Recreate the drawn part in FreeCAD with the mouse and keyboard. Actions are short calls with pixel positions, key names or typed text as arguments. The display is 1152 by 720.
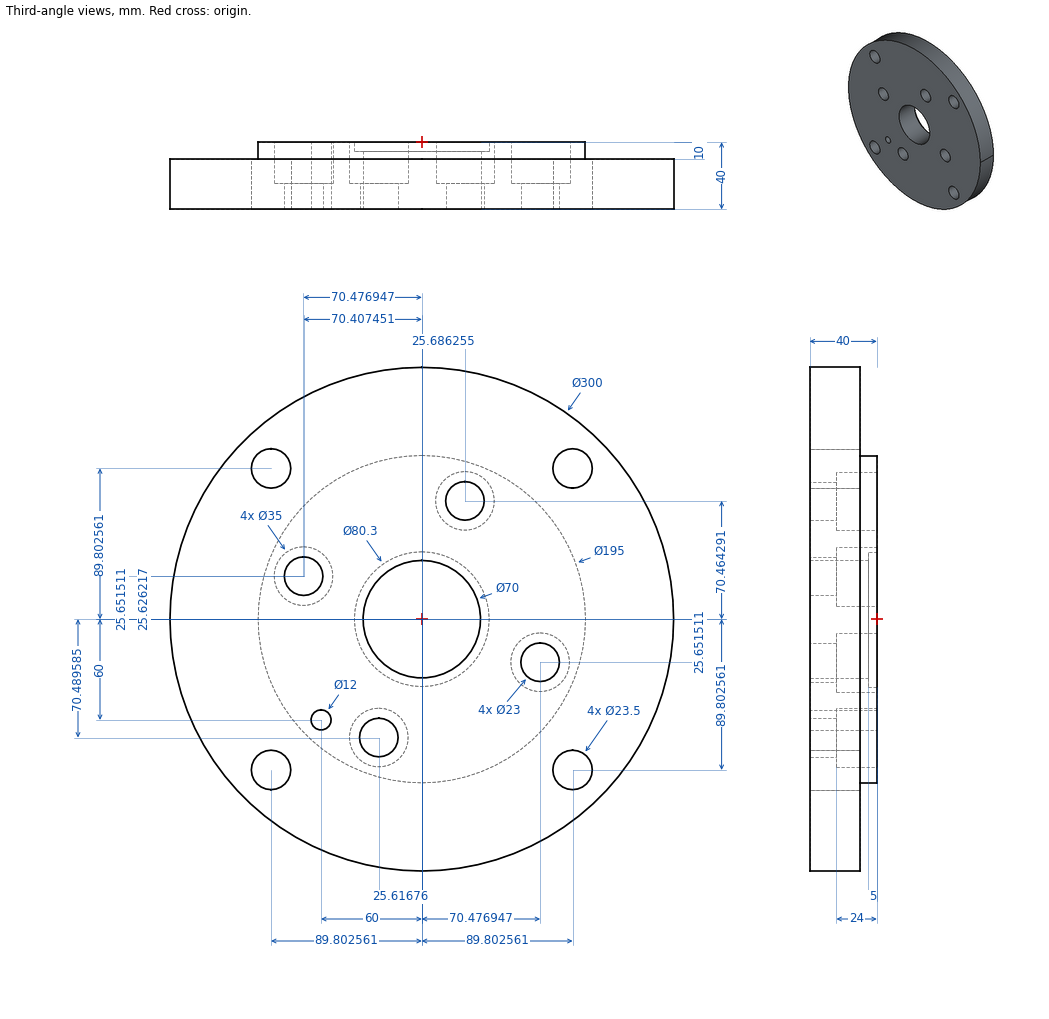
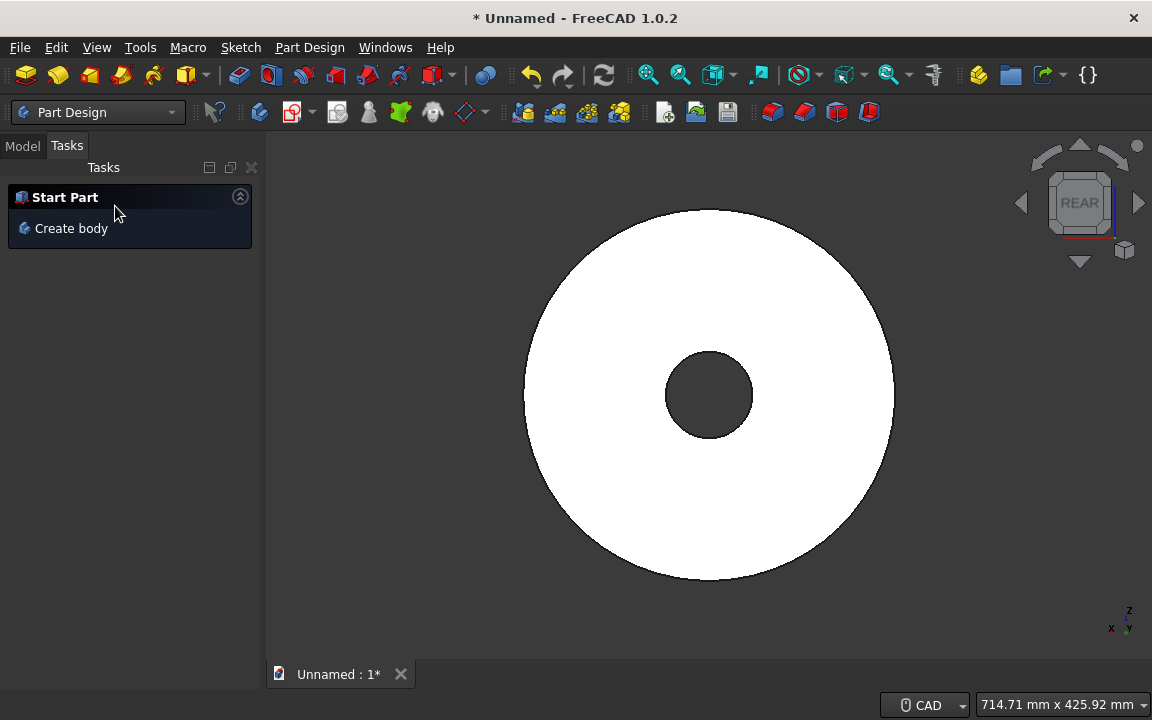
click(656, 500)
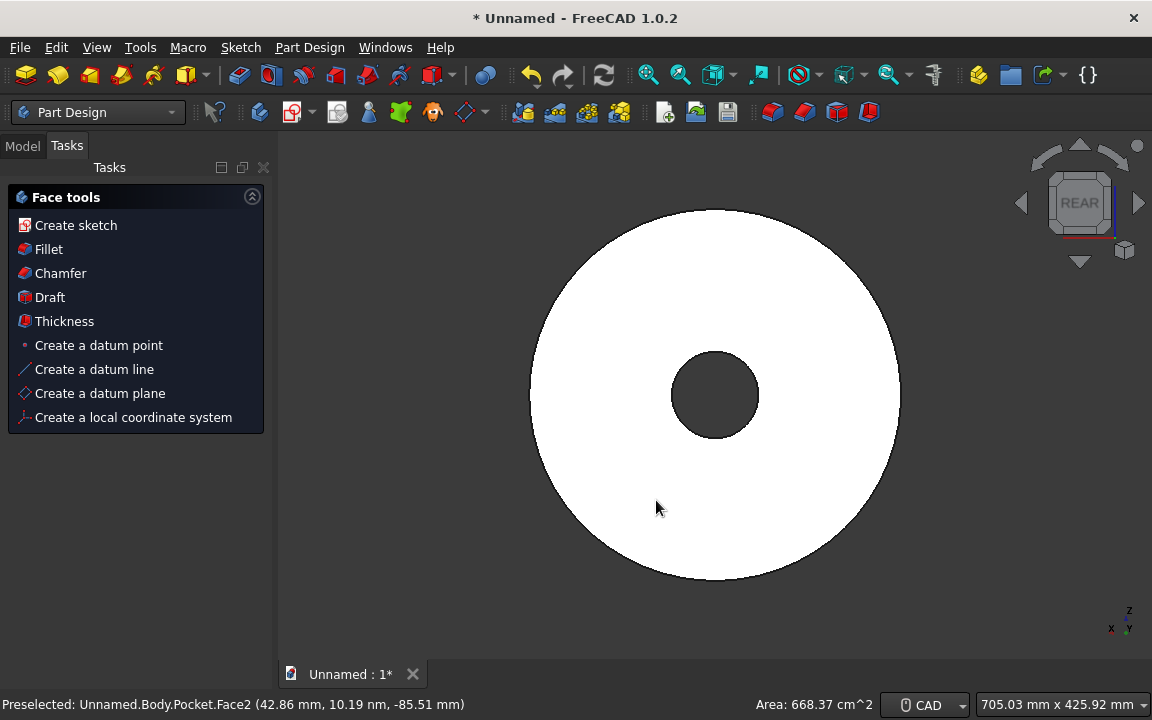
click(292, 112)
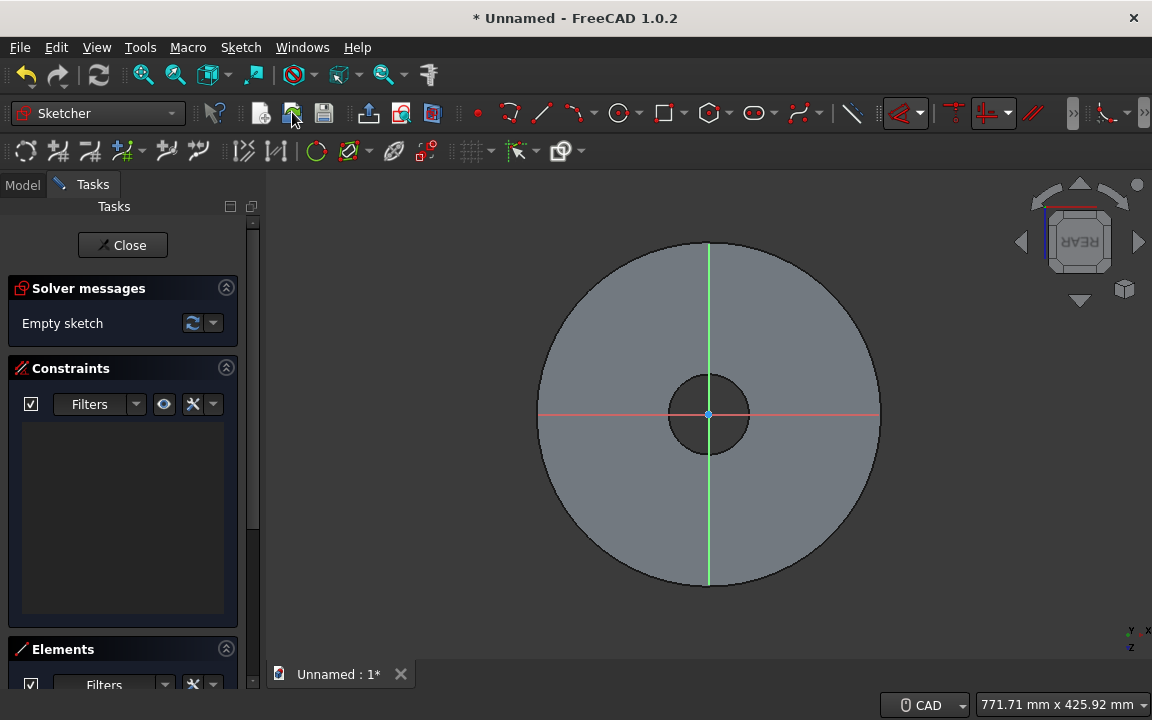
scroll(738, 414, up, 6)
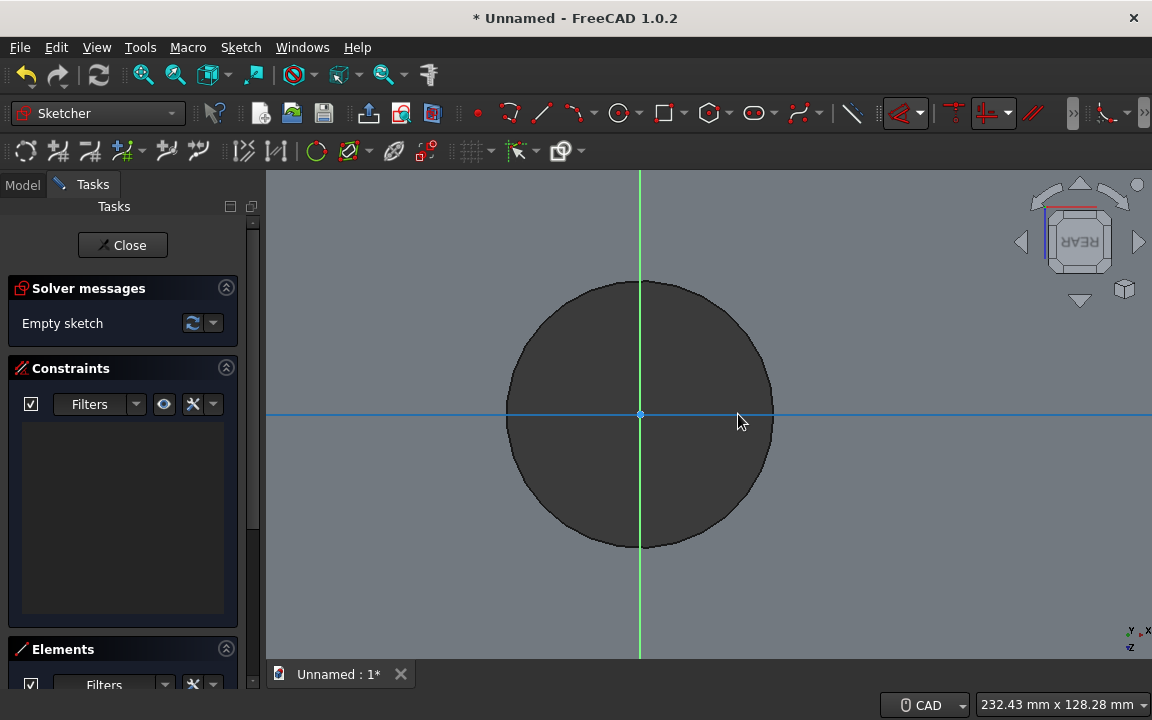
click(620, 114)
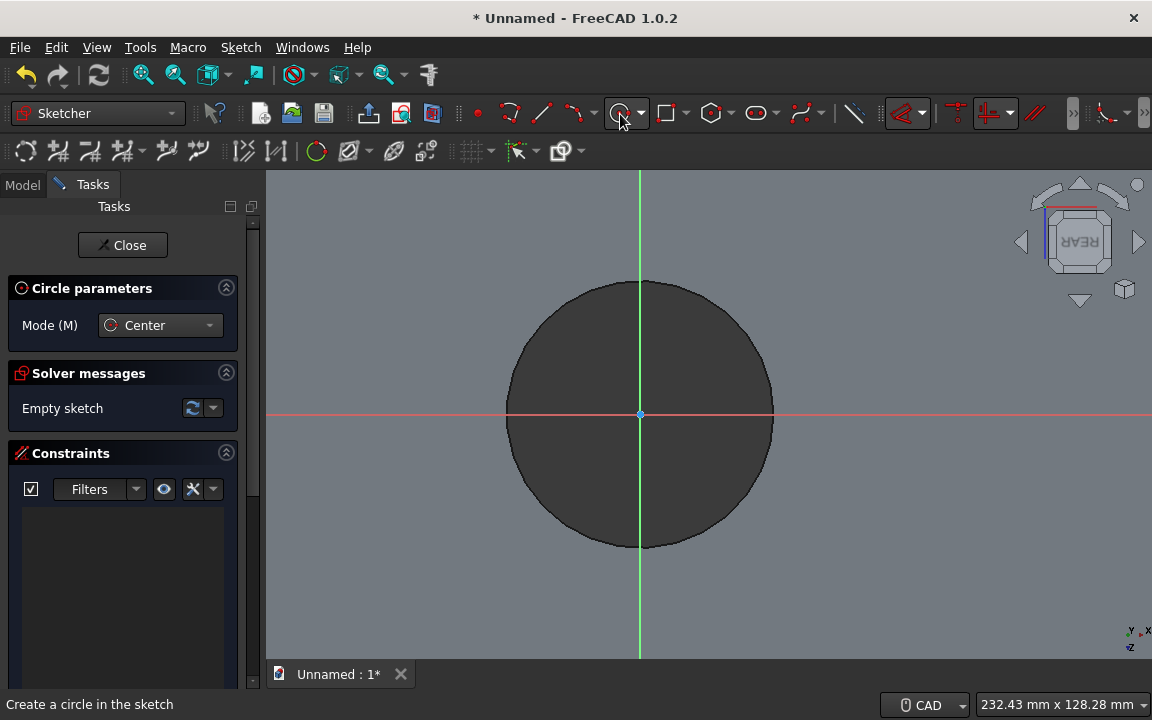
click(640, 414)
move(748, 306)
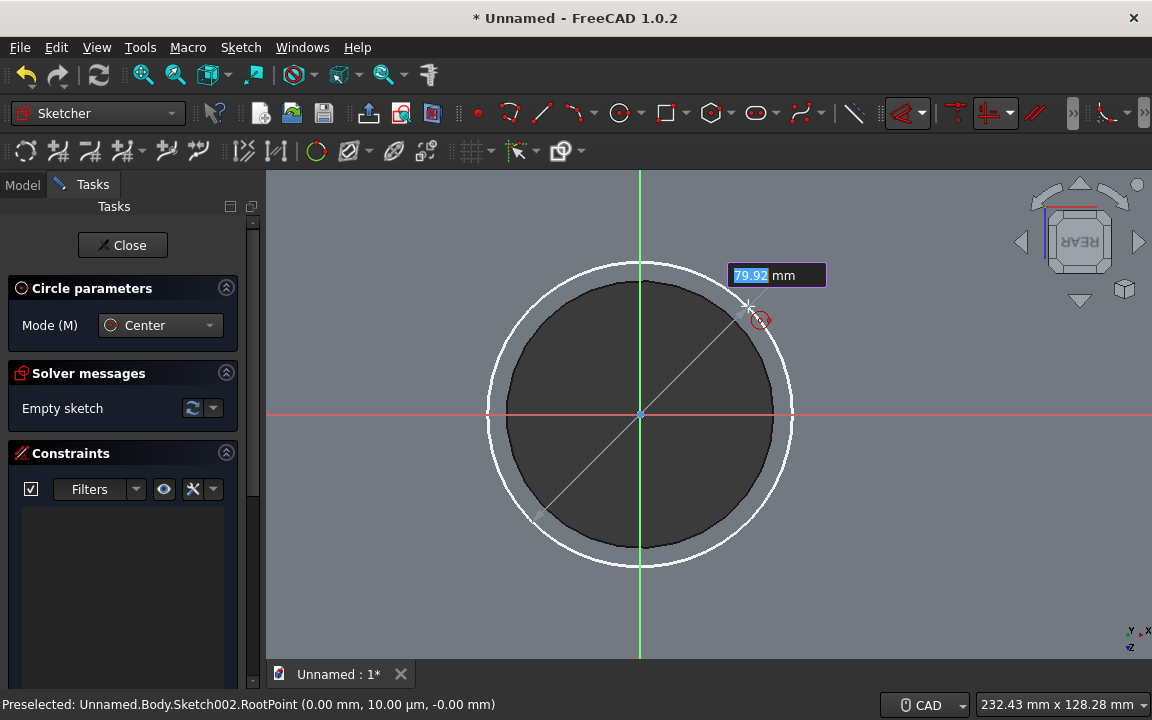
text(80.3)
key(Return)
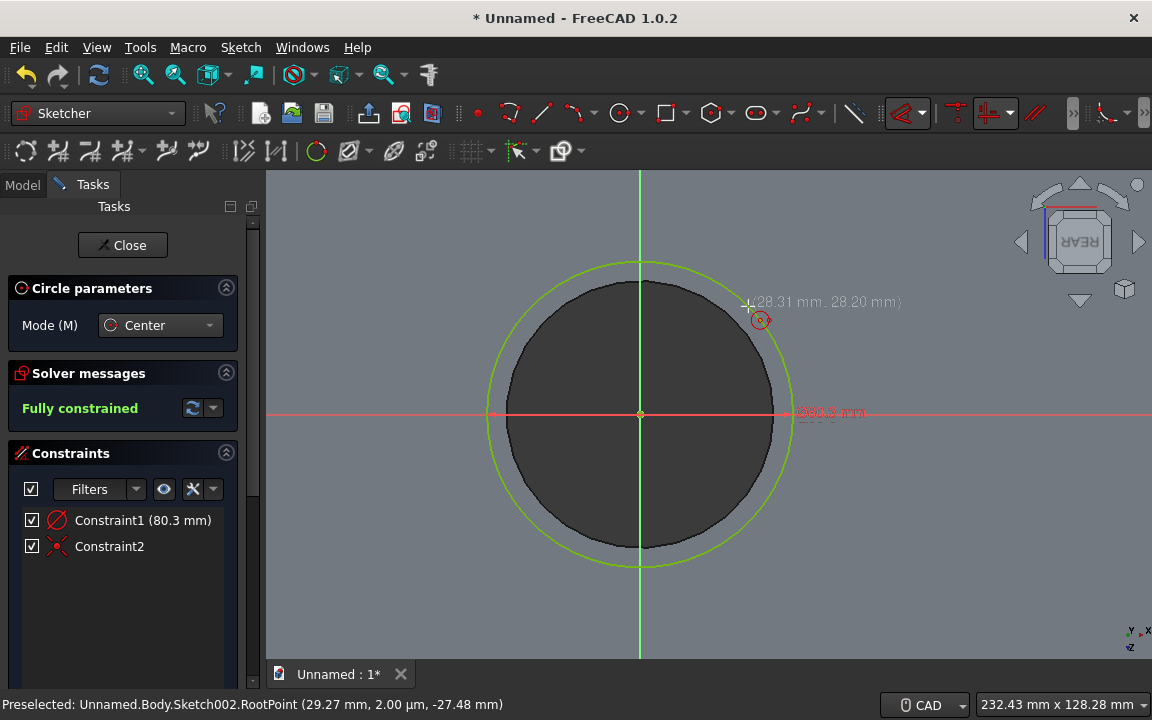
click(640, 414)
move(734, 320)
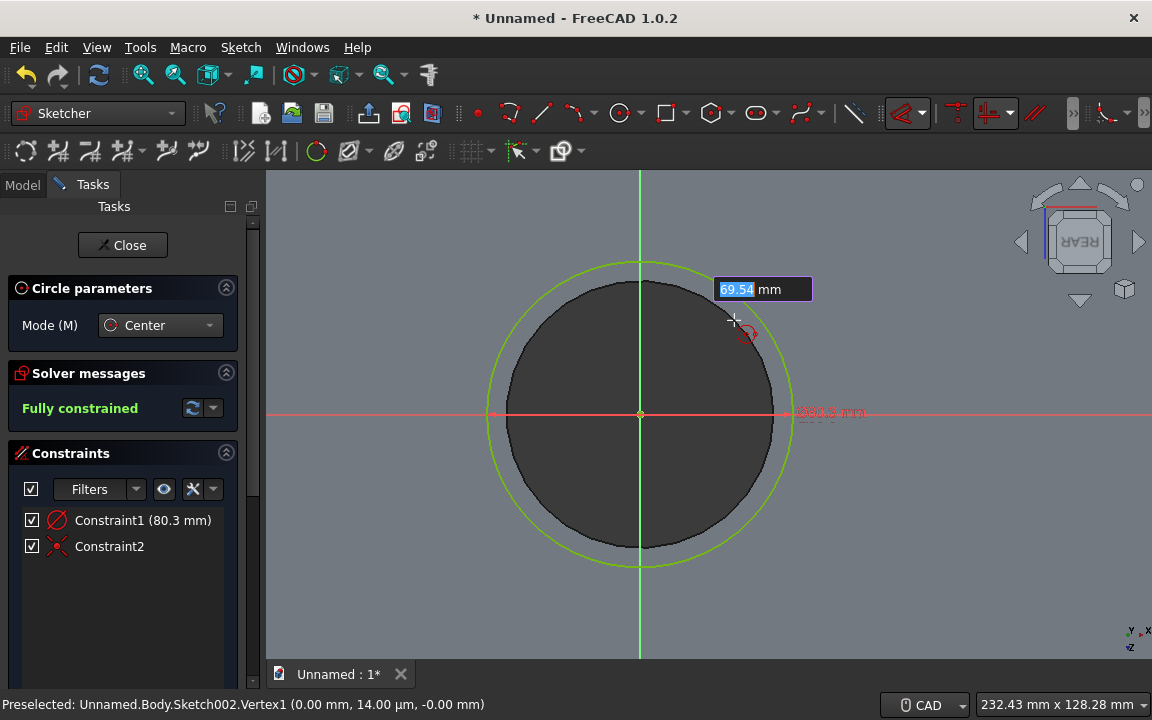
text(70)
key(Return)
key(Escape)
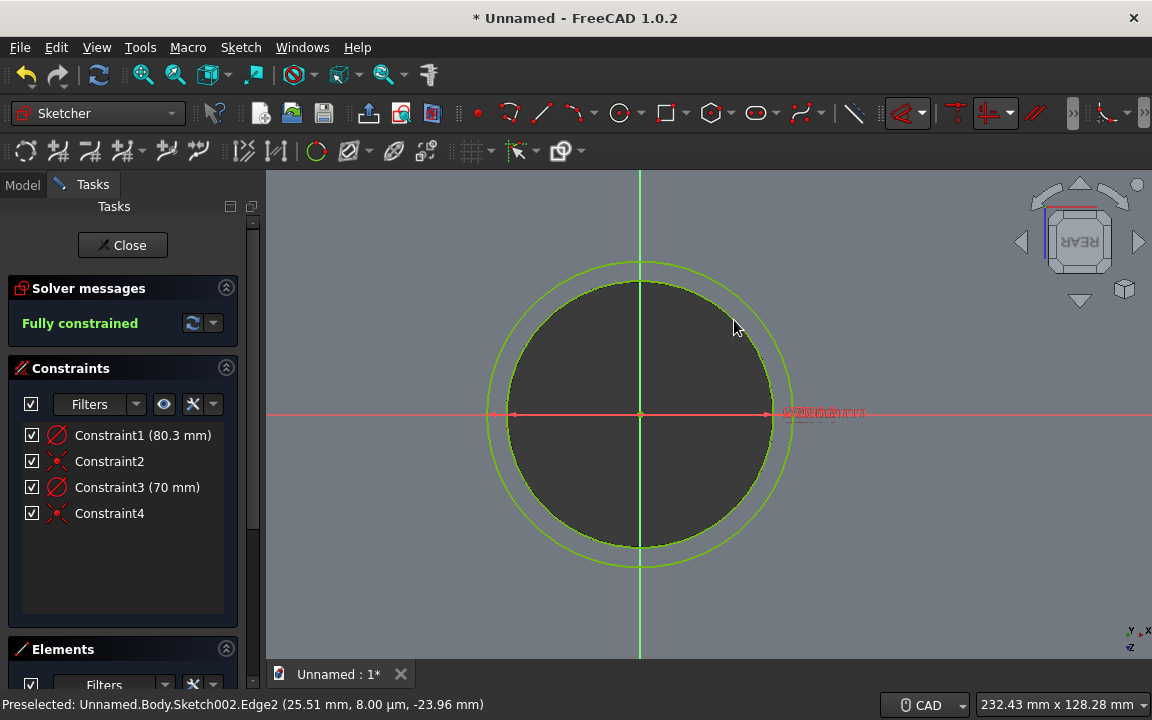
click(123, 245)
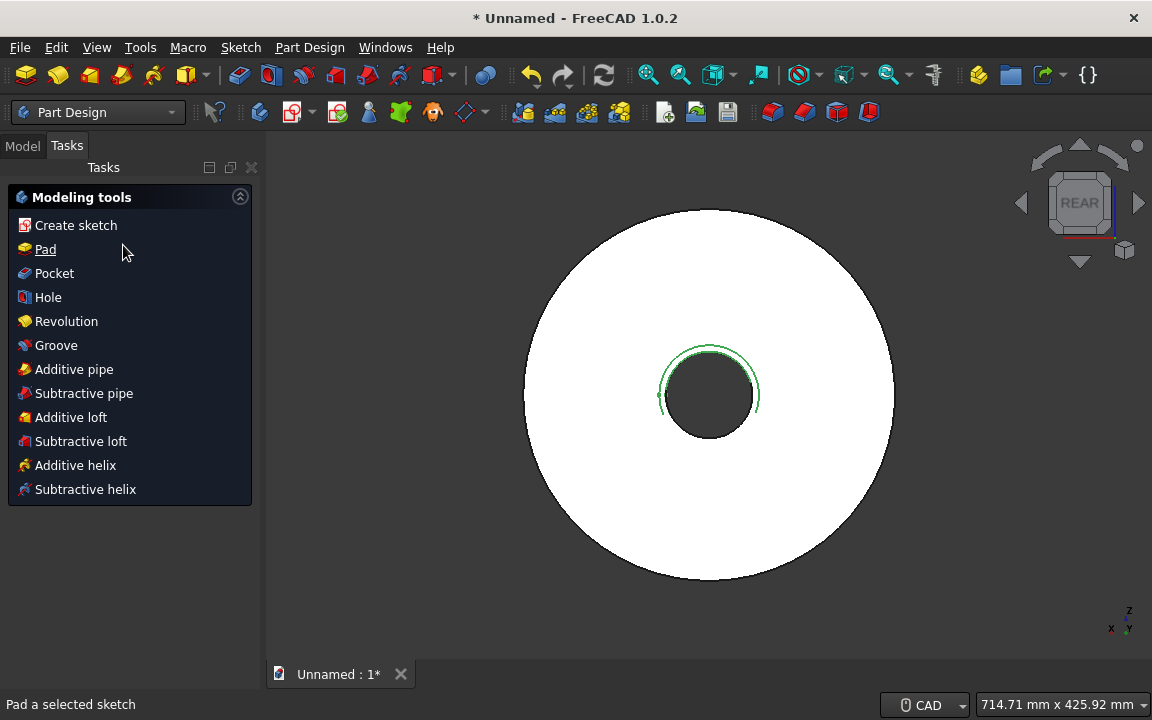
click(240, 76)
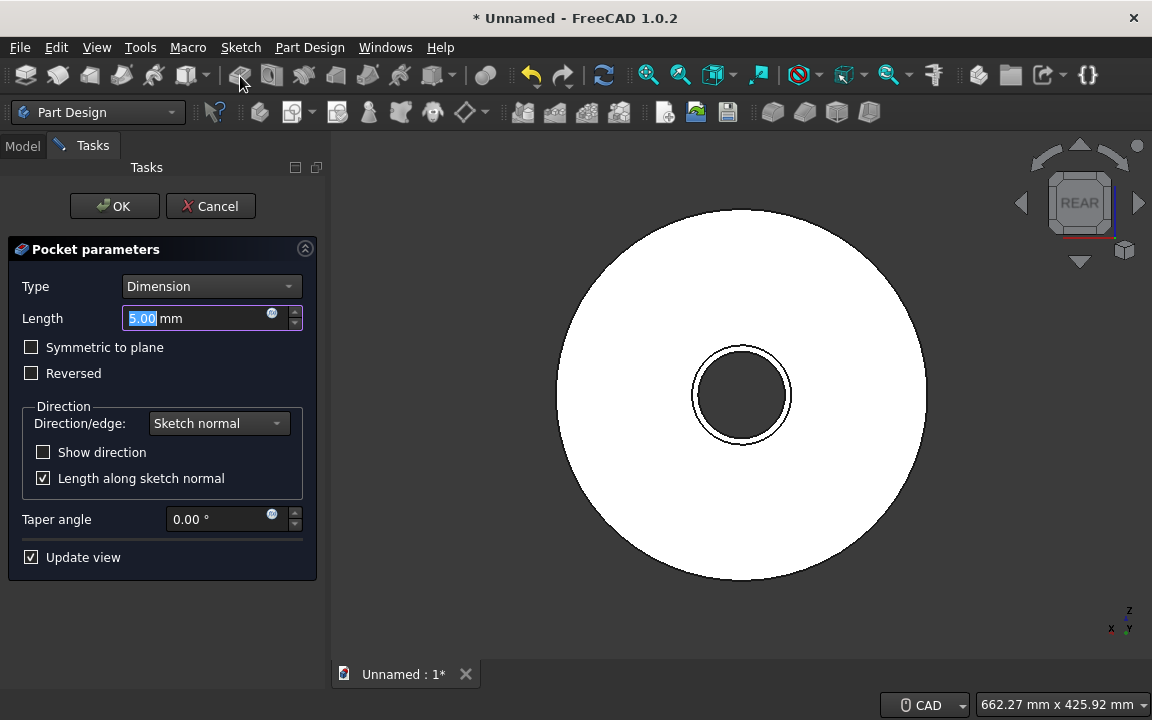
text(5)
key(Tab)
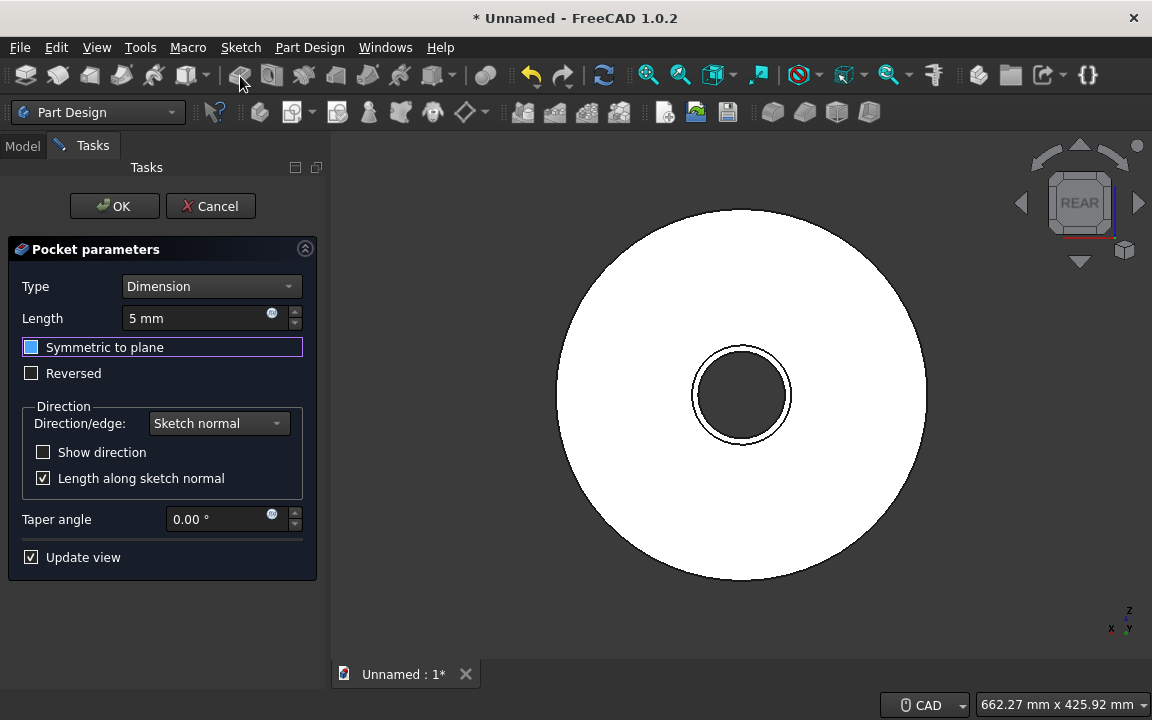
click(115, 206)